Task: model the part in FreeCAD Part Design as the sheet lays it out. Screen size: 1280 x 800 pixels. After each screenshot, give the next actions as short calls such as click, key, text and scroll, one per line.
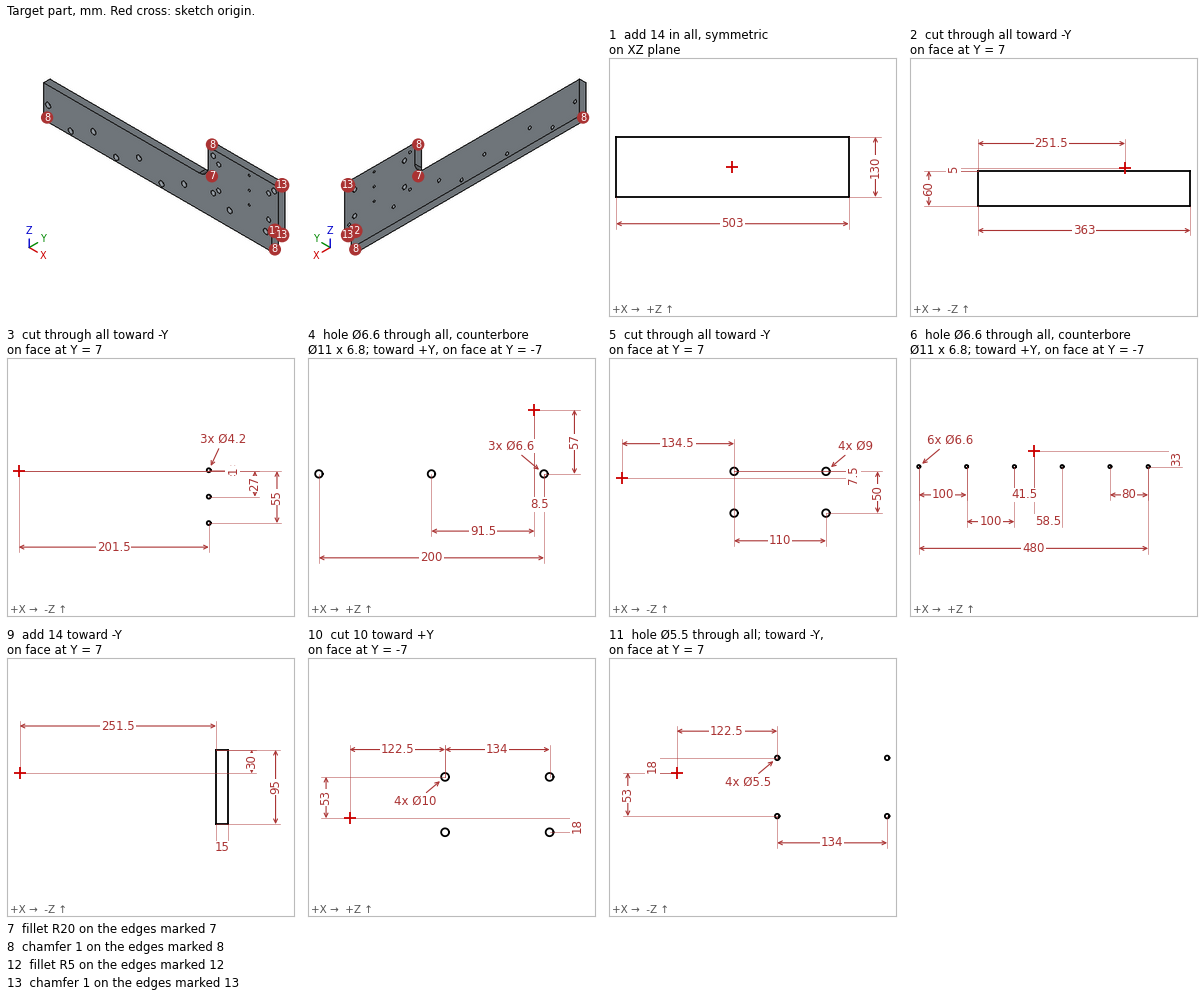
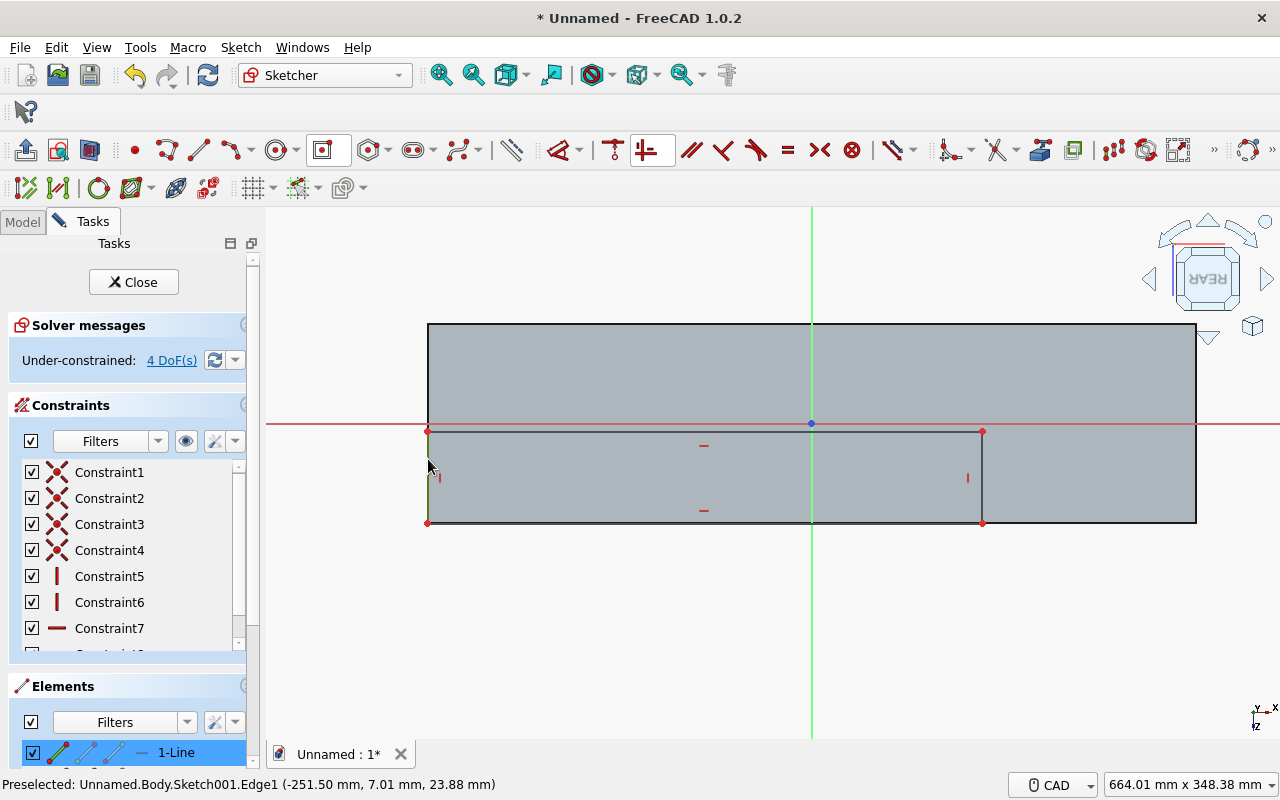
click(582, 150)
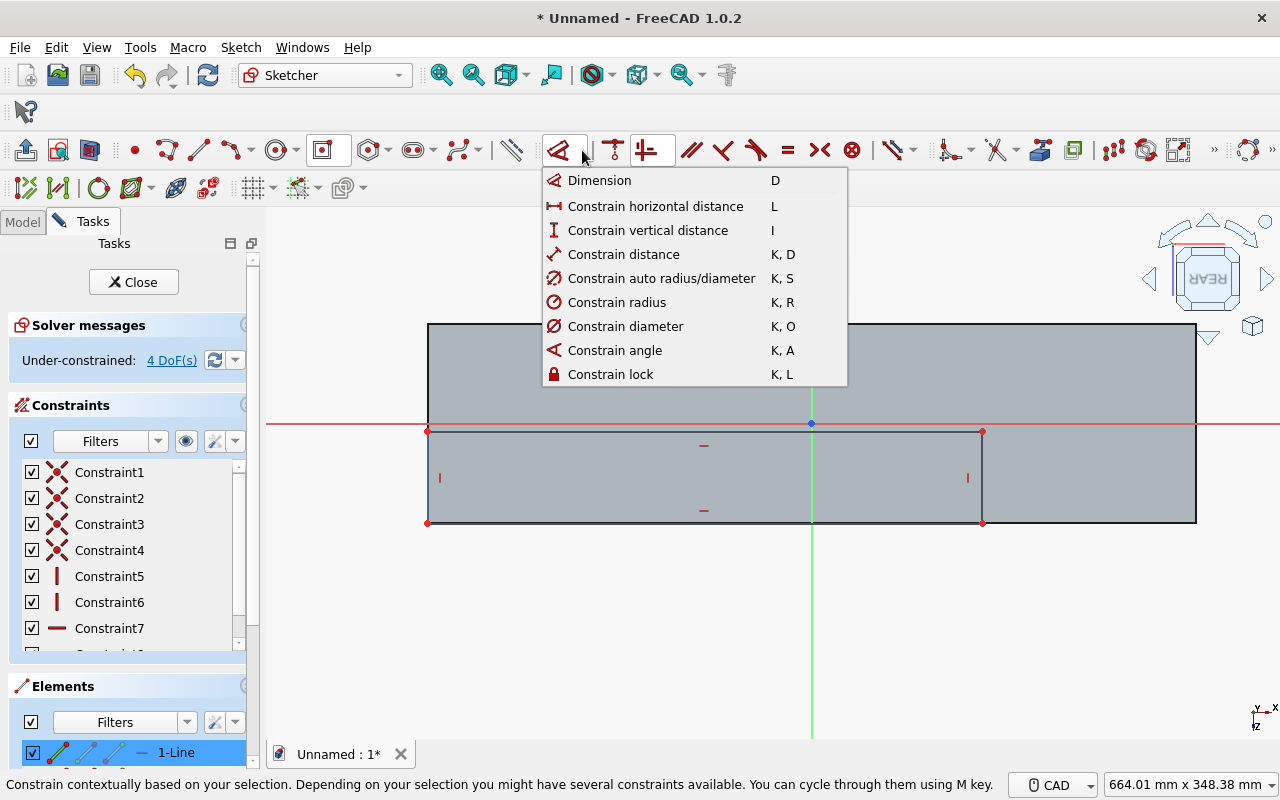
click(695, 230)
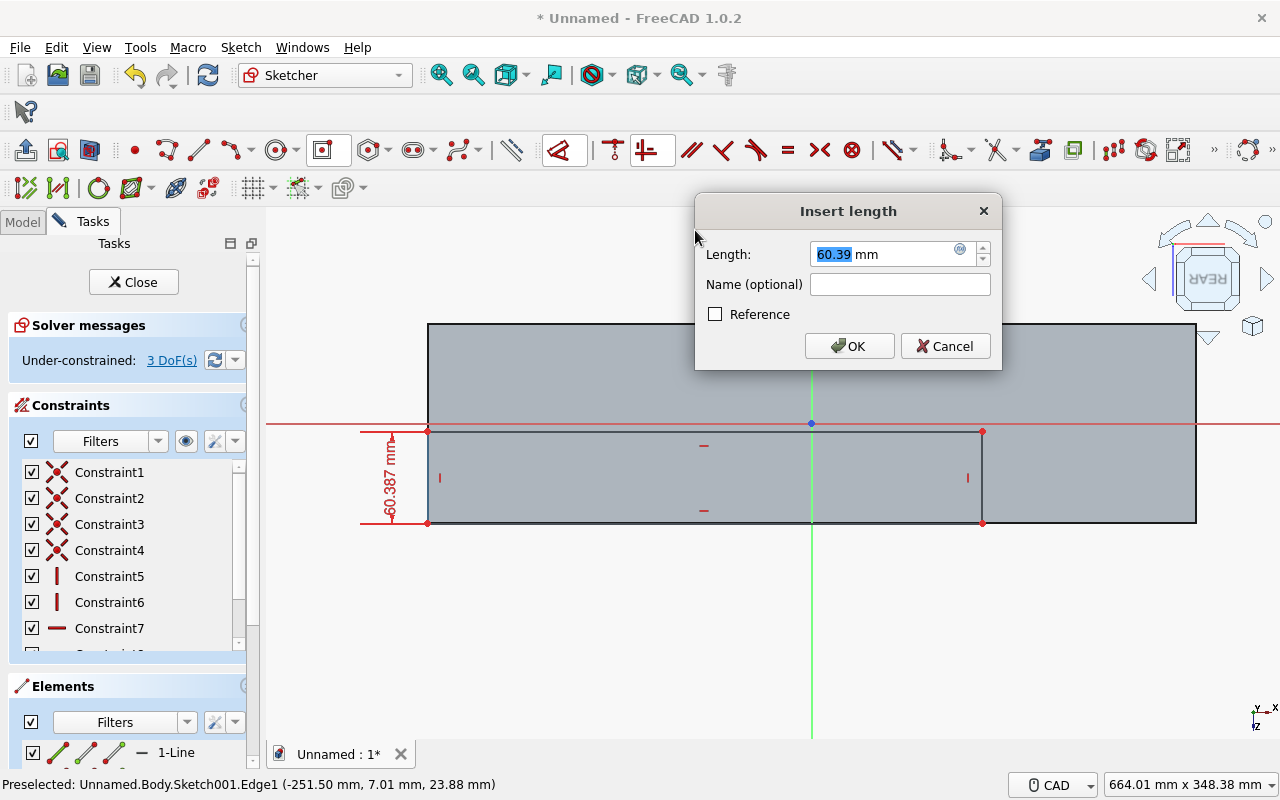
text(60)
key(Return)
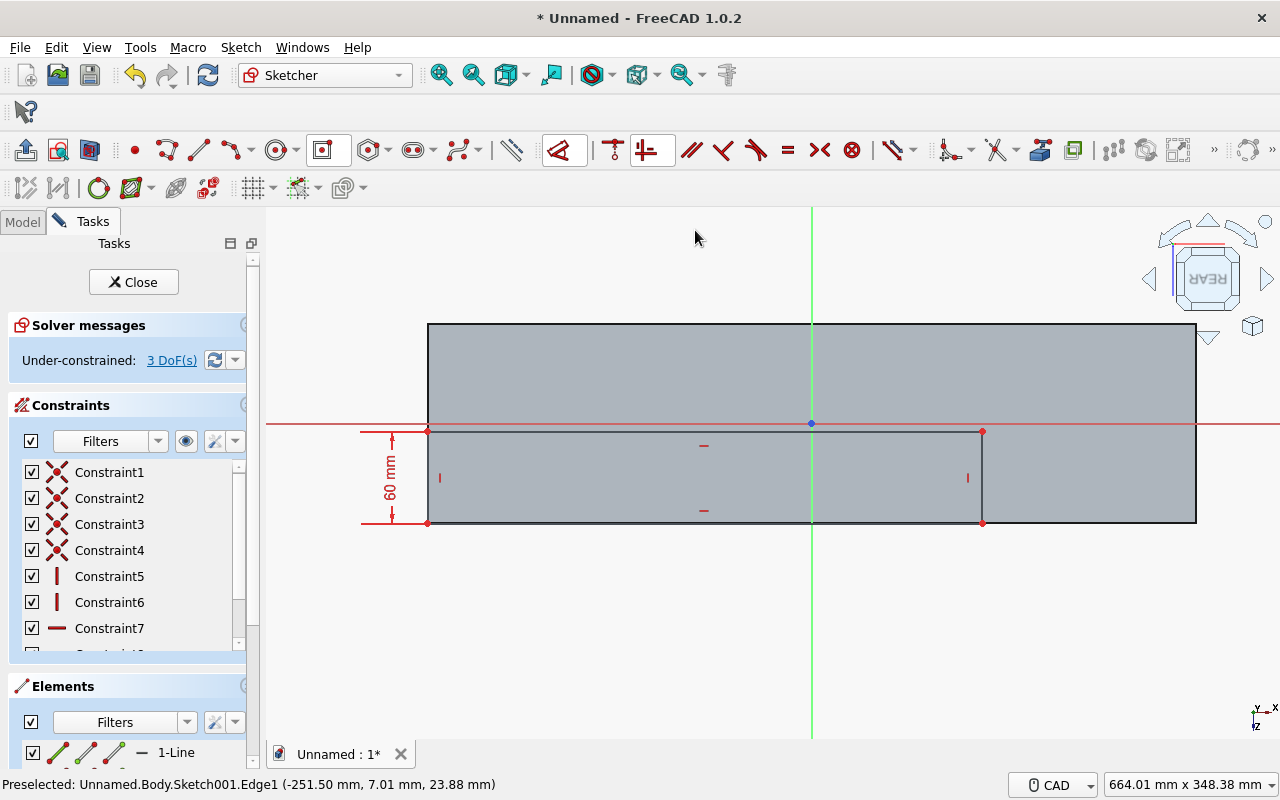
scroll(428, 432, up, 9)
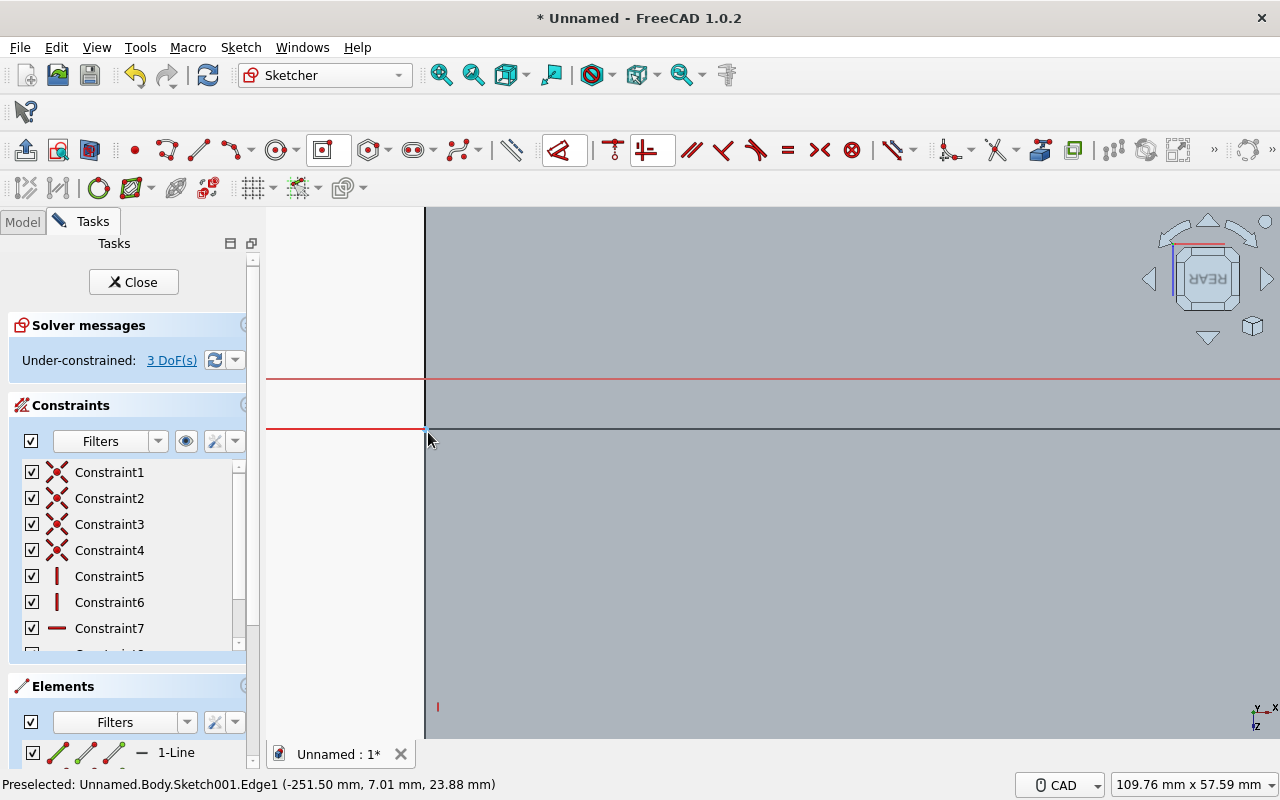
click(425, 429)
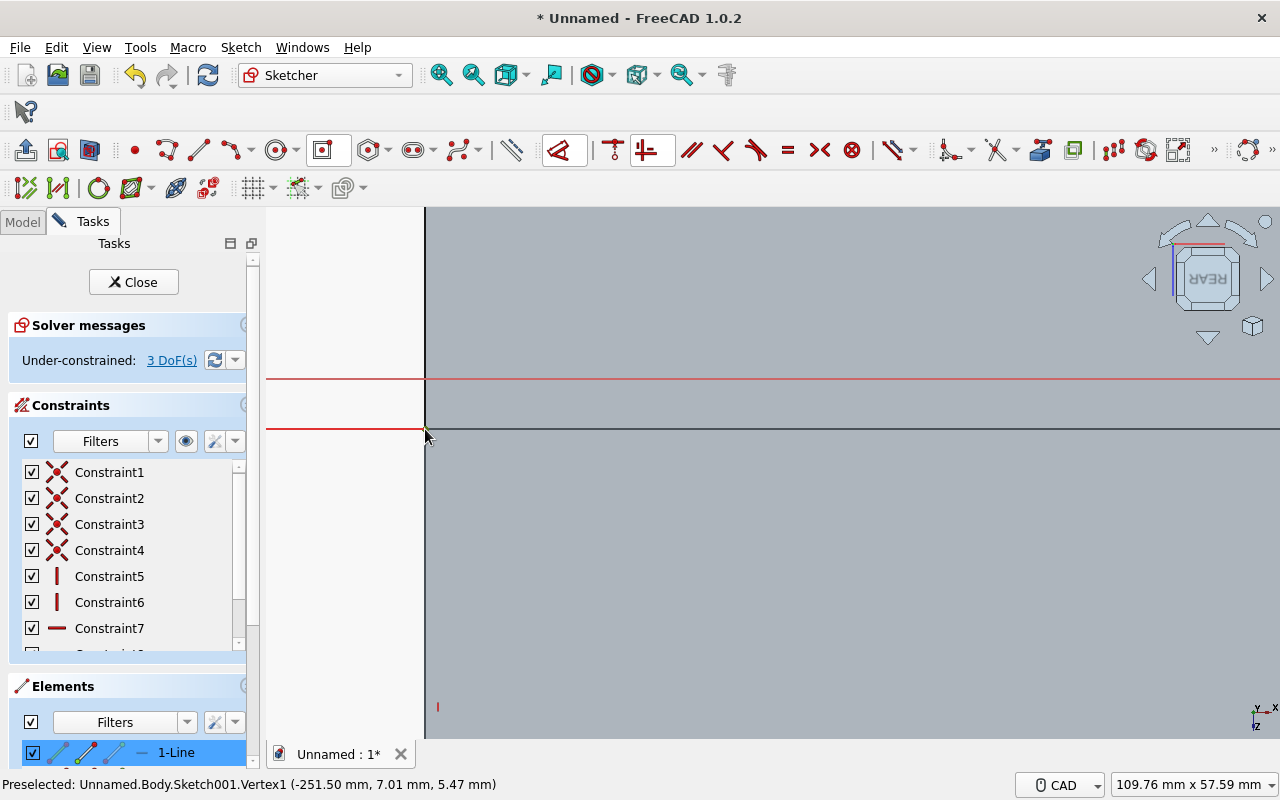
key(i)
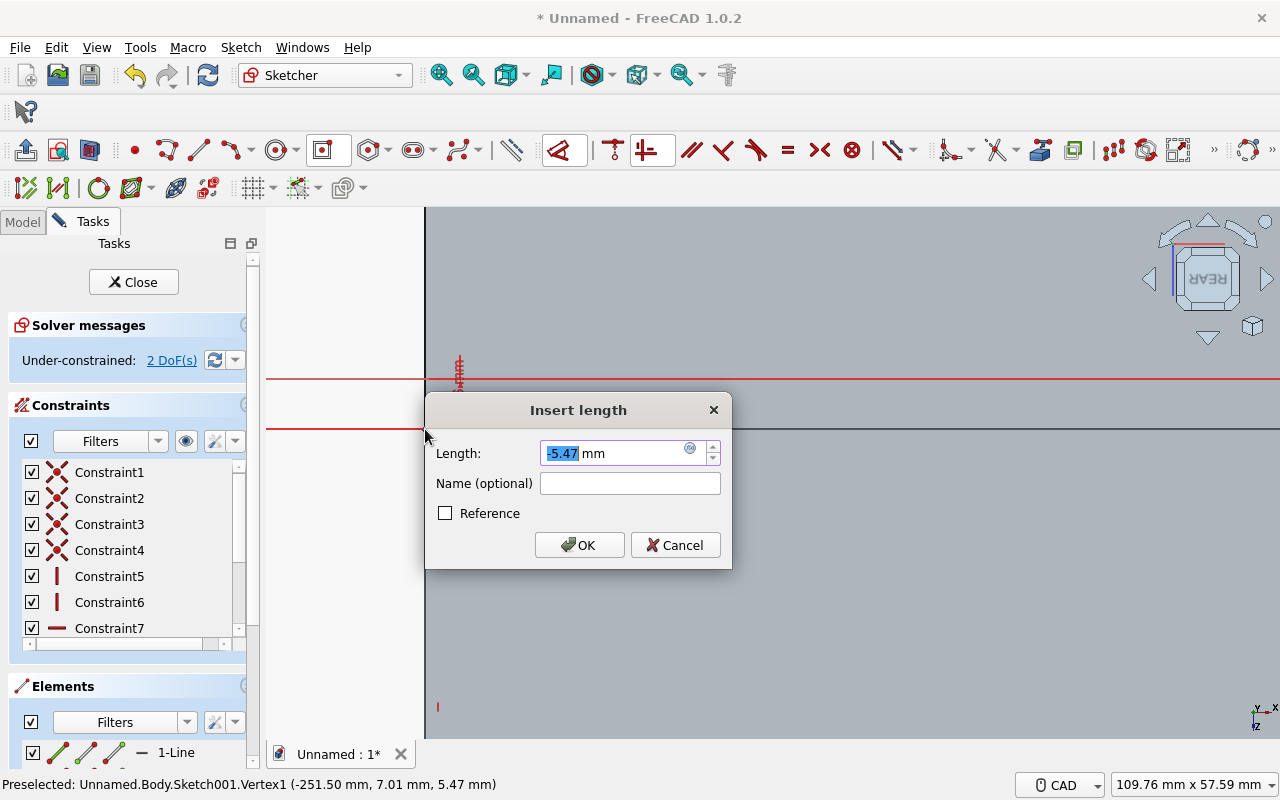
text(-5)
key(Return)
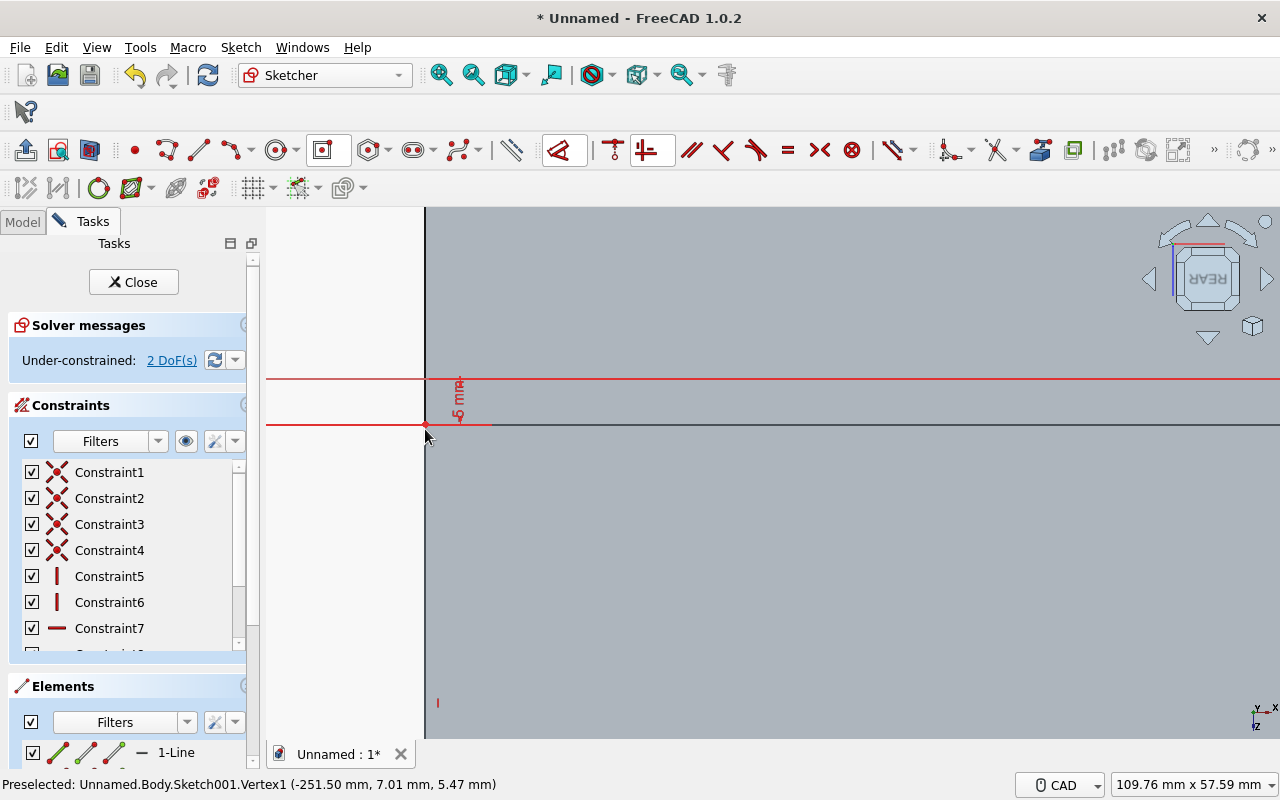
scroll(428, 432, down, 9)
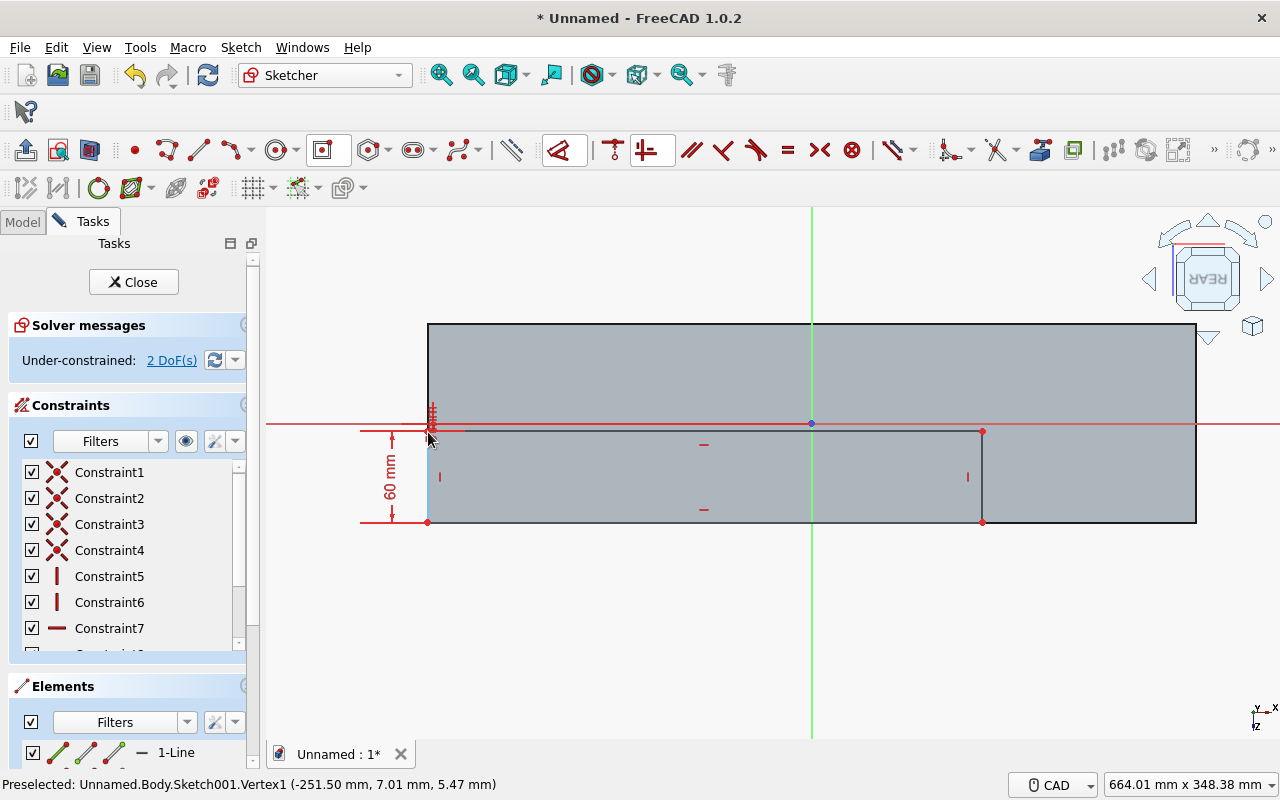
click(594, 523)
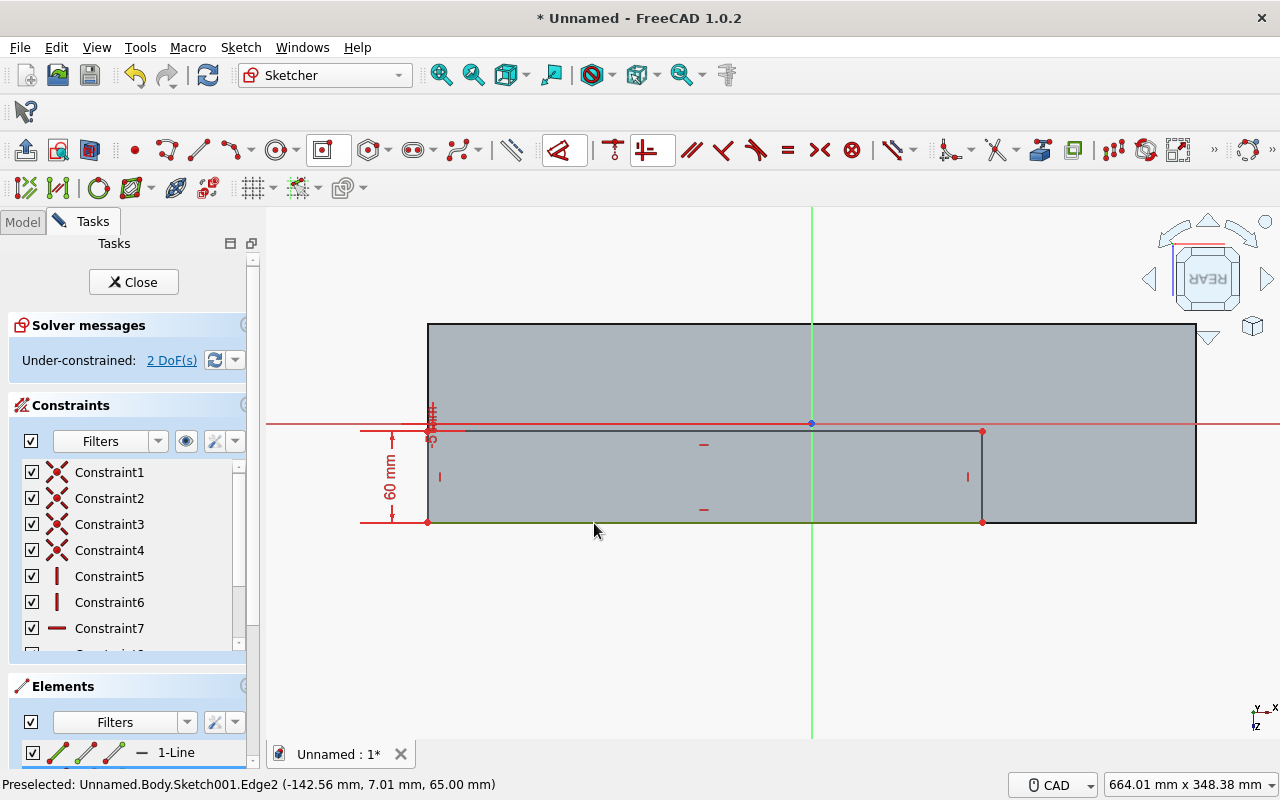
key(l)